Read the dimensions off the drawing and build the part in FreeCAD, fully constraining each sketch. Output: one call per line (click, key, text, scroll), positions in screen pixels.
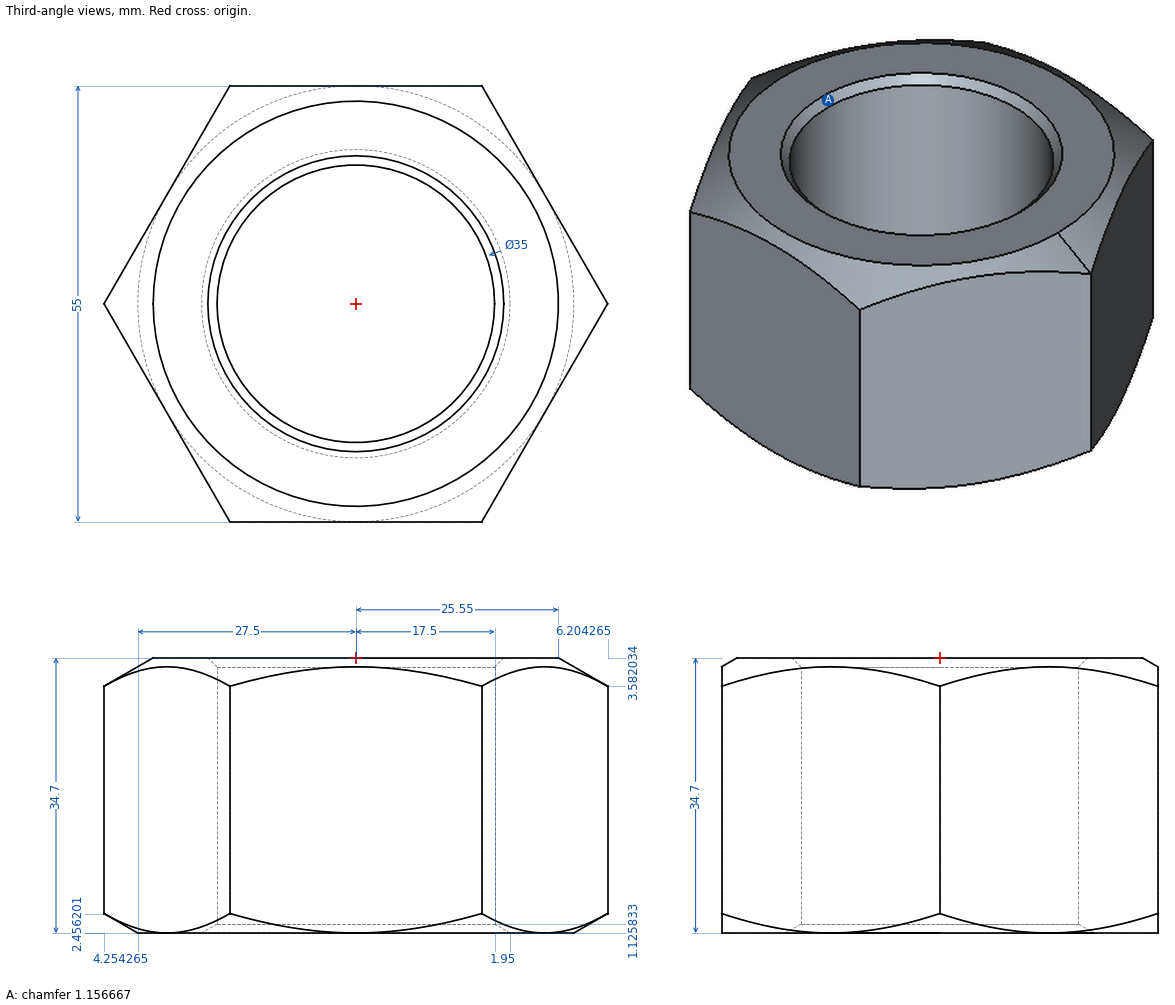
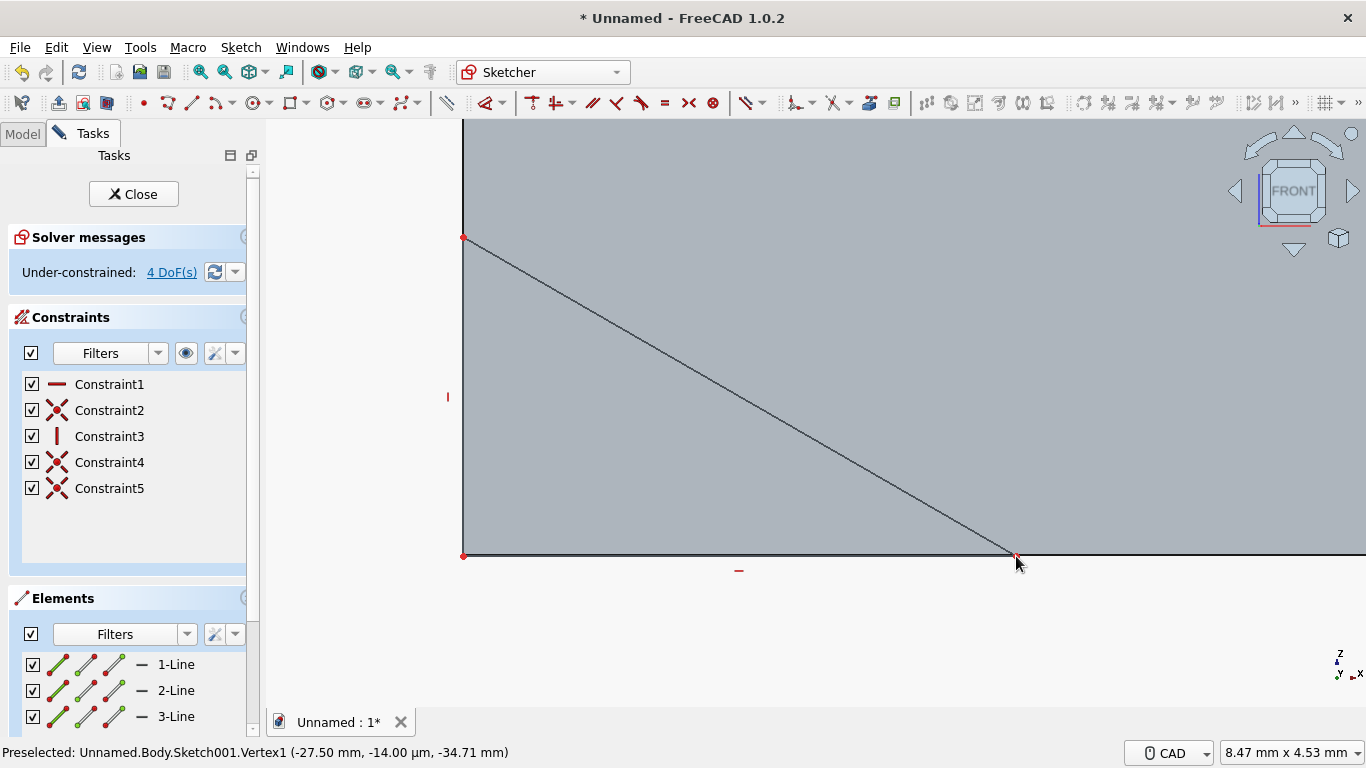
click(1016, 556)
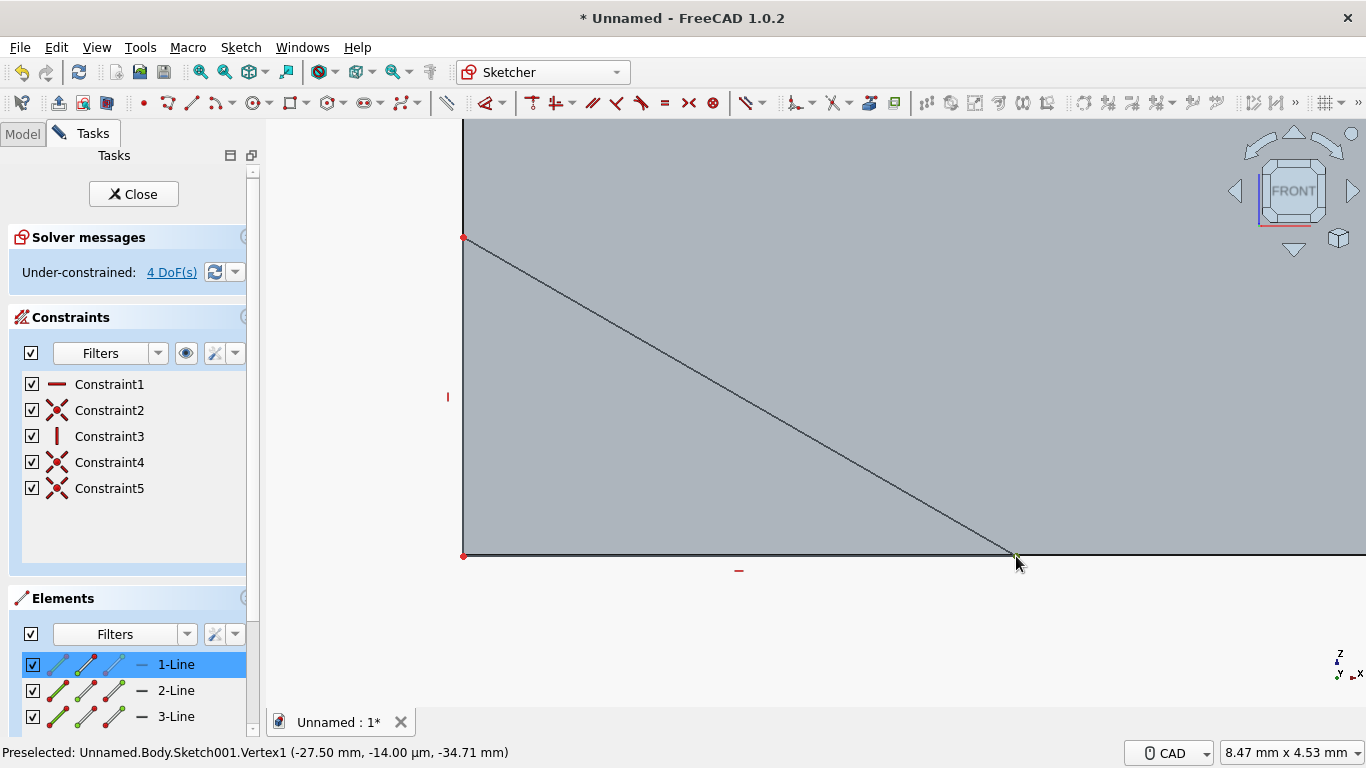
click(504, 104)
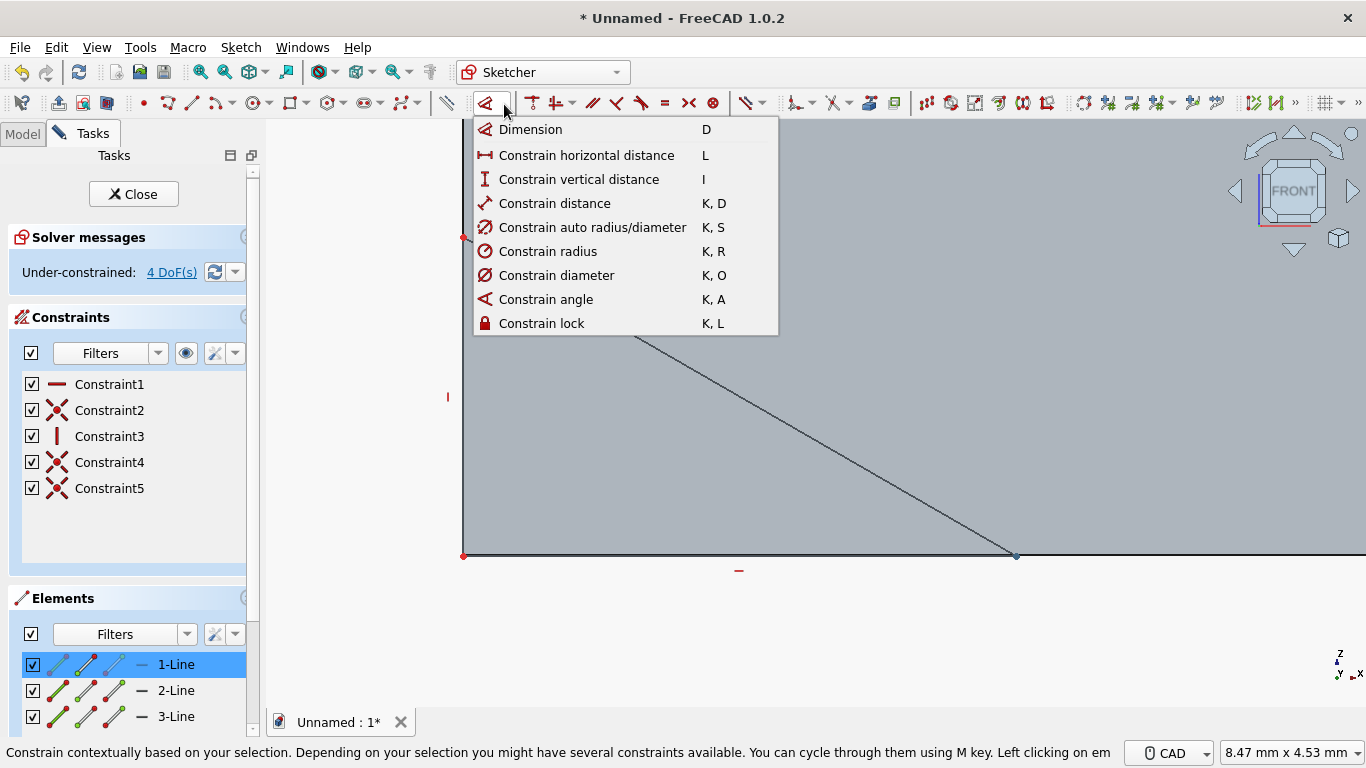
click(626, 155)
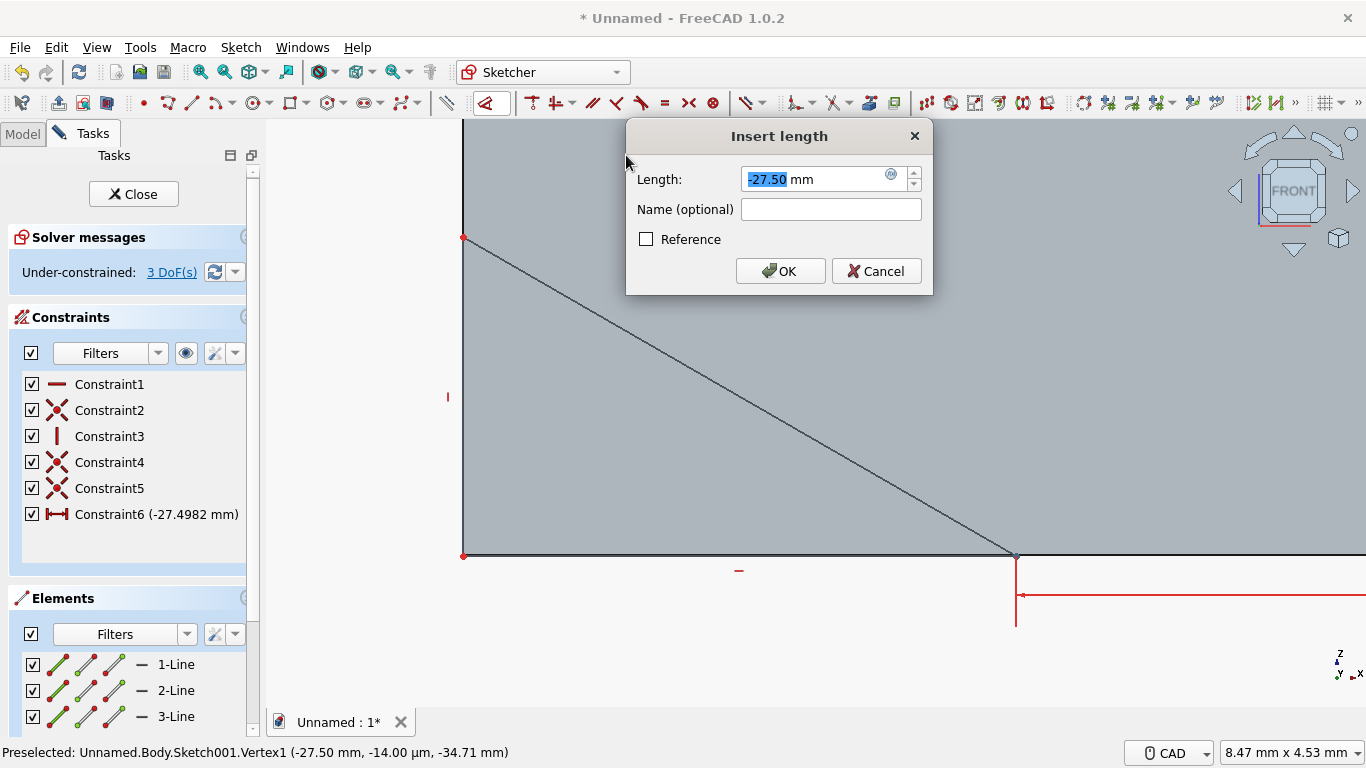
text(-27.5)
key(Return)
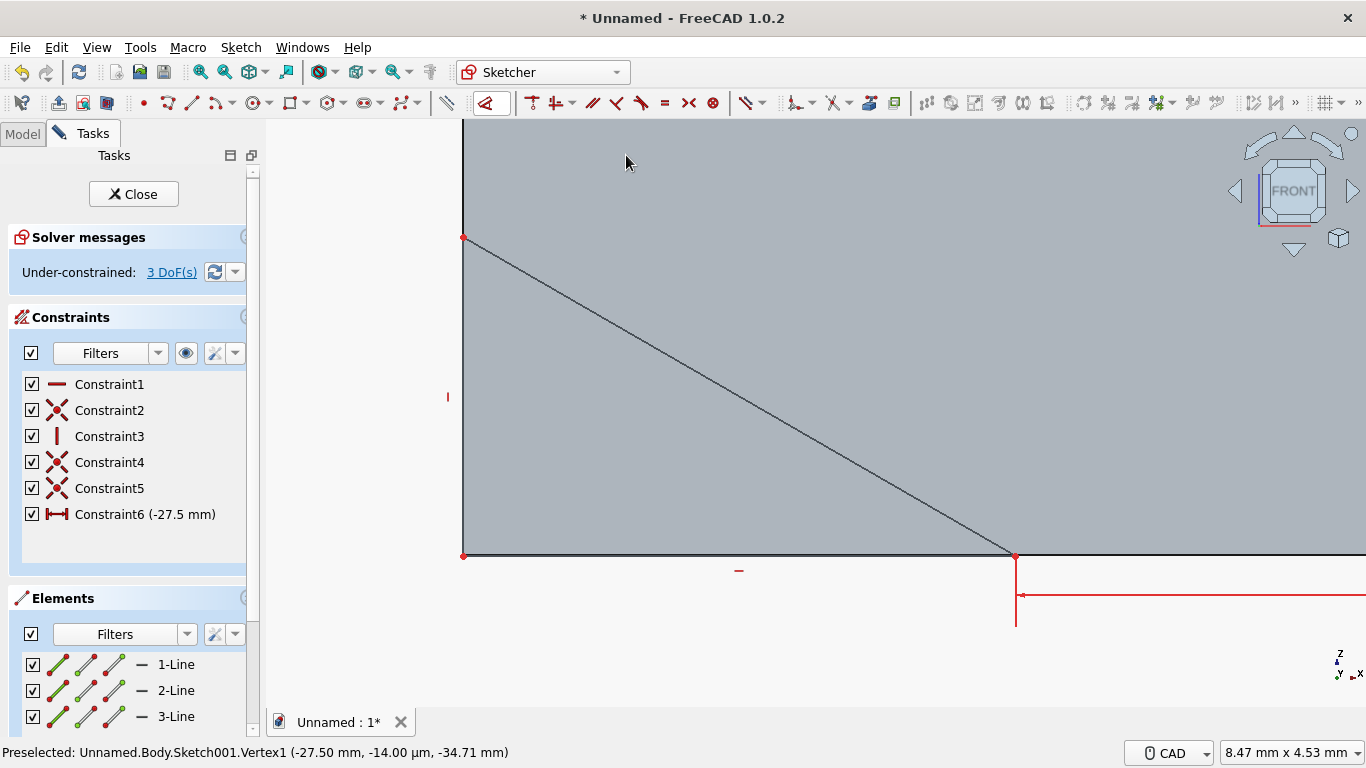
click(1016, 556)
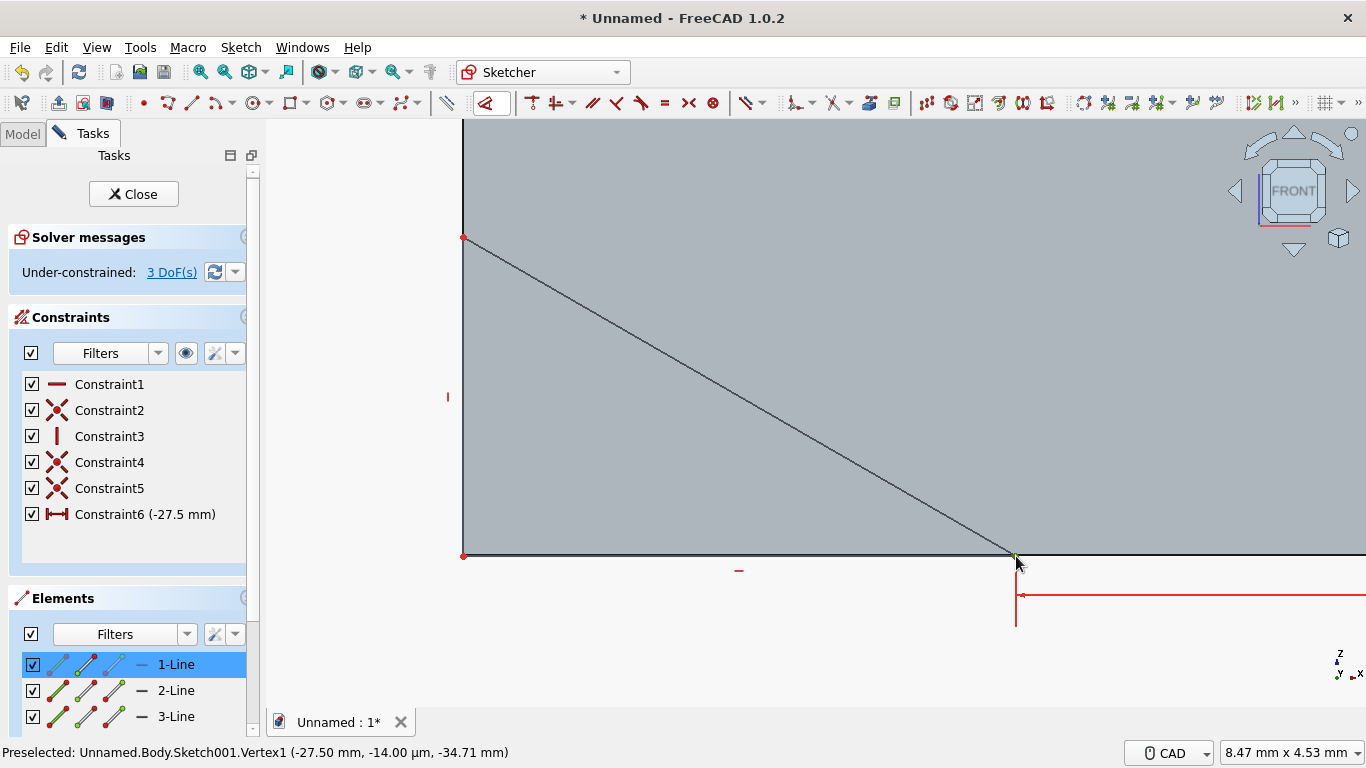
click(504, 104)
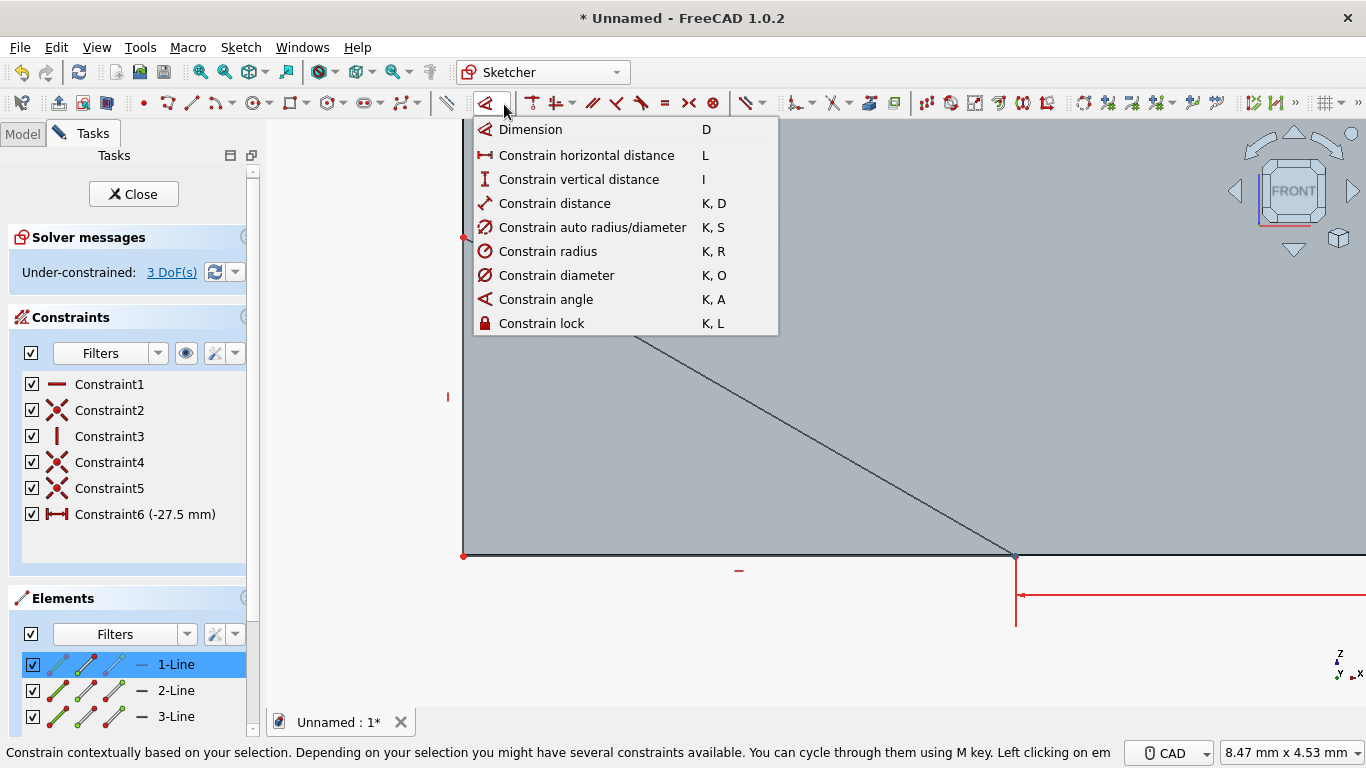
click(626, 179)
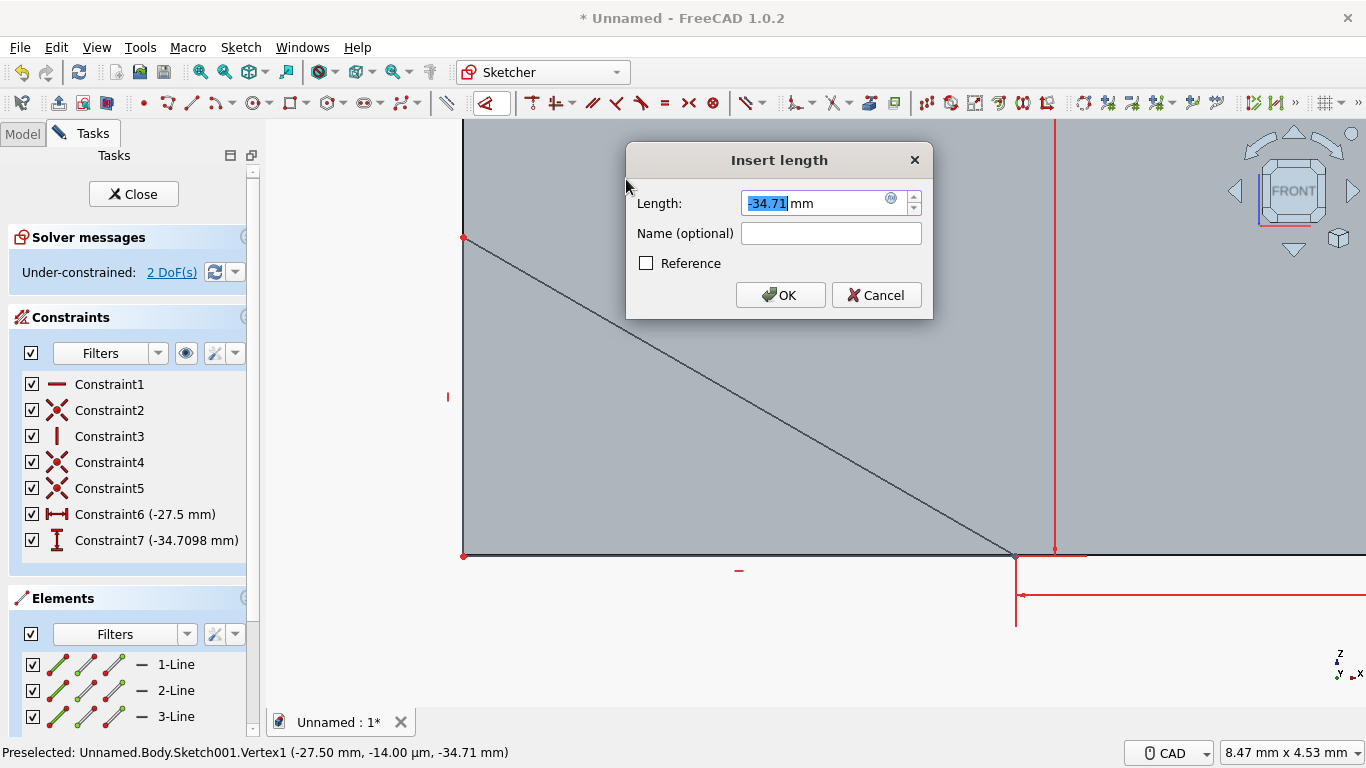
text(-34.7)
key(Return)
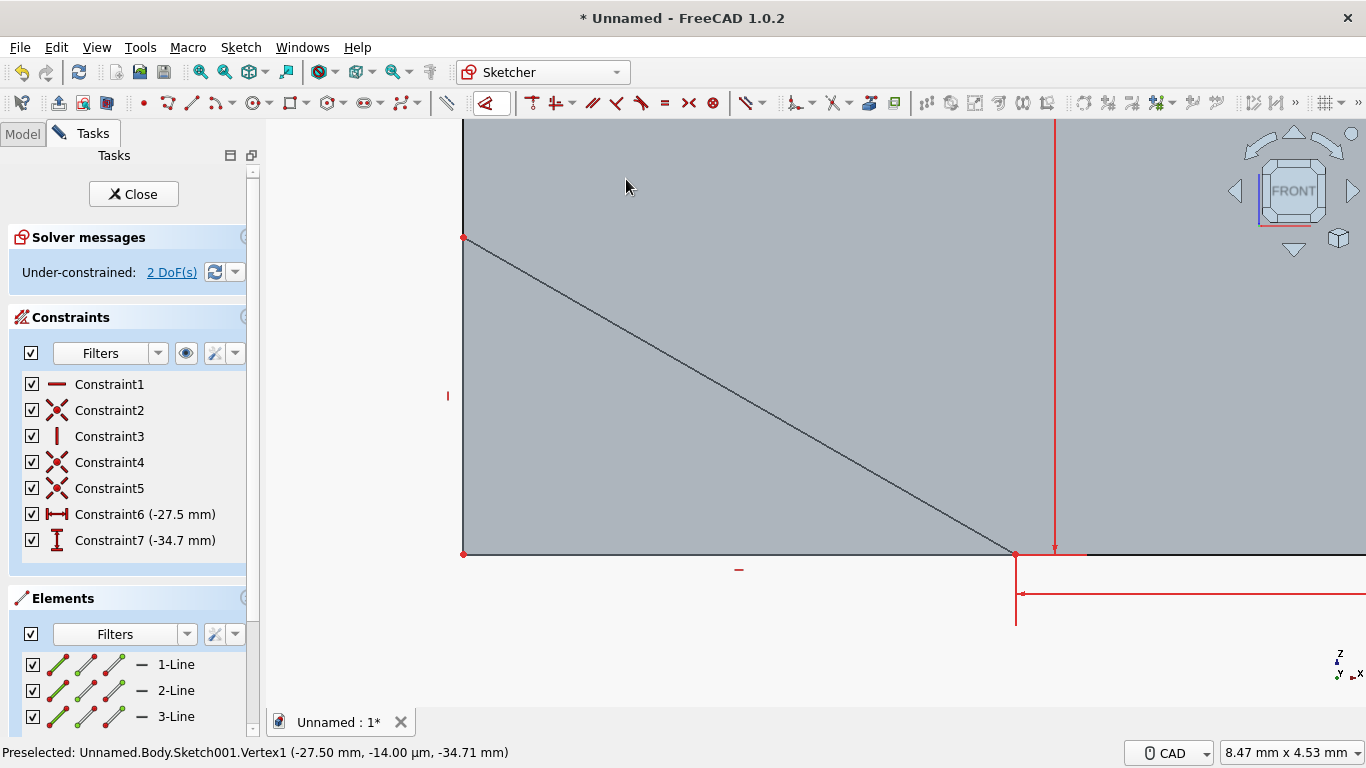
click(850, 555)